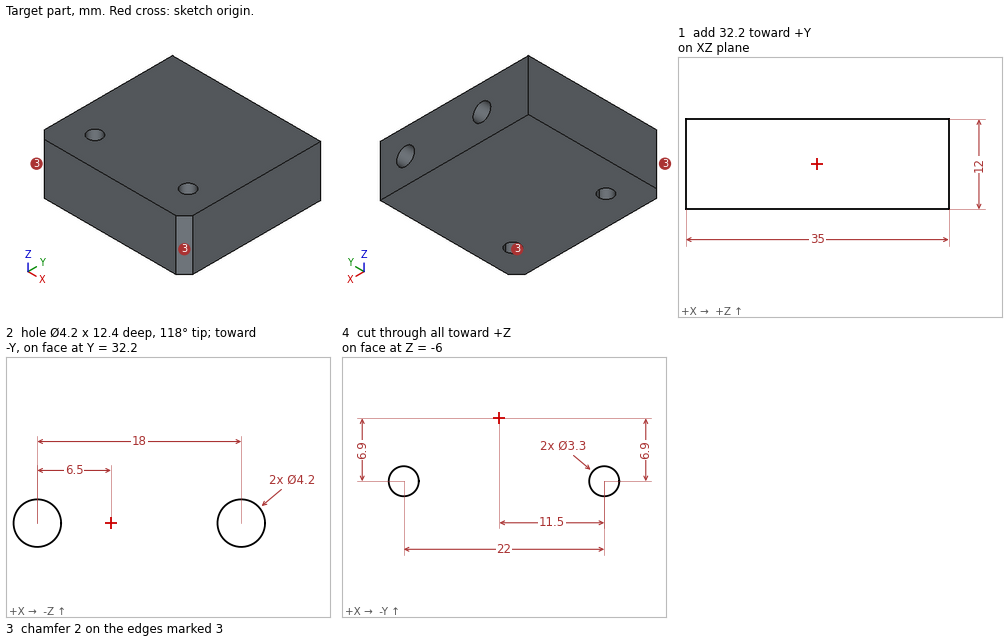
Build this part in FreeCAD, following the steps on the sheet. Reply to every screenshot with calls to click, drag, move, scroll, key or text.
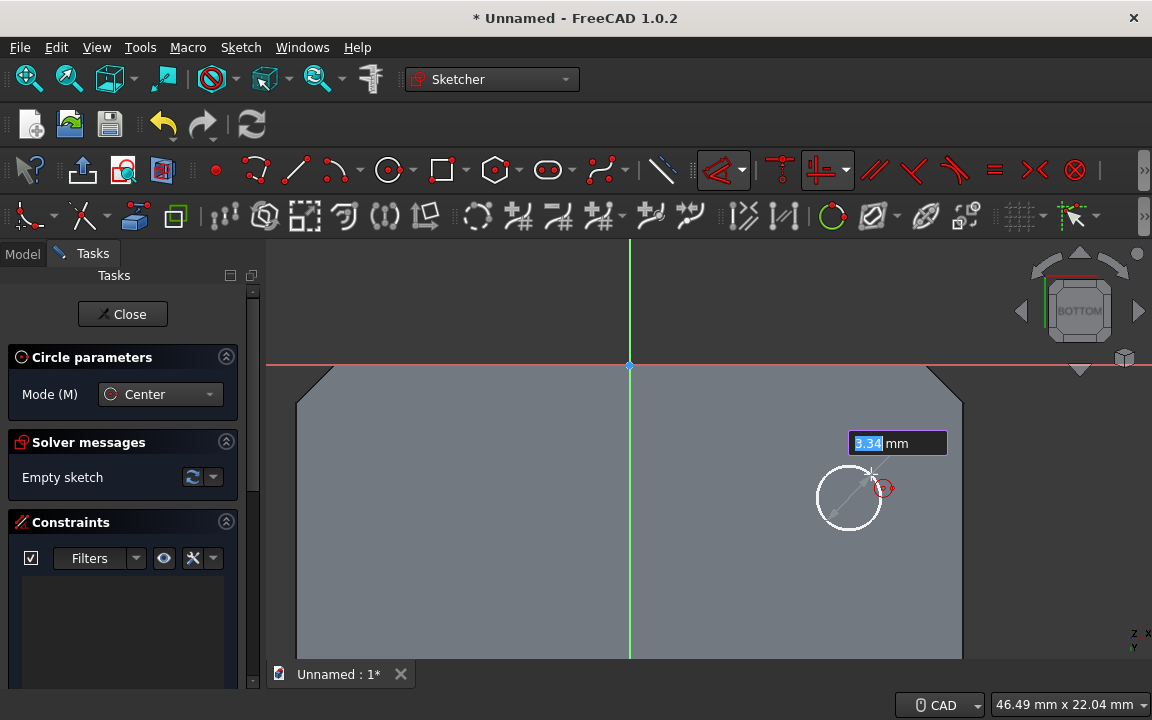
text(3.3)
key(Return)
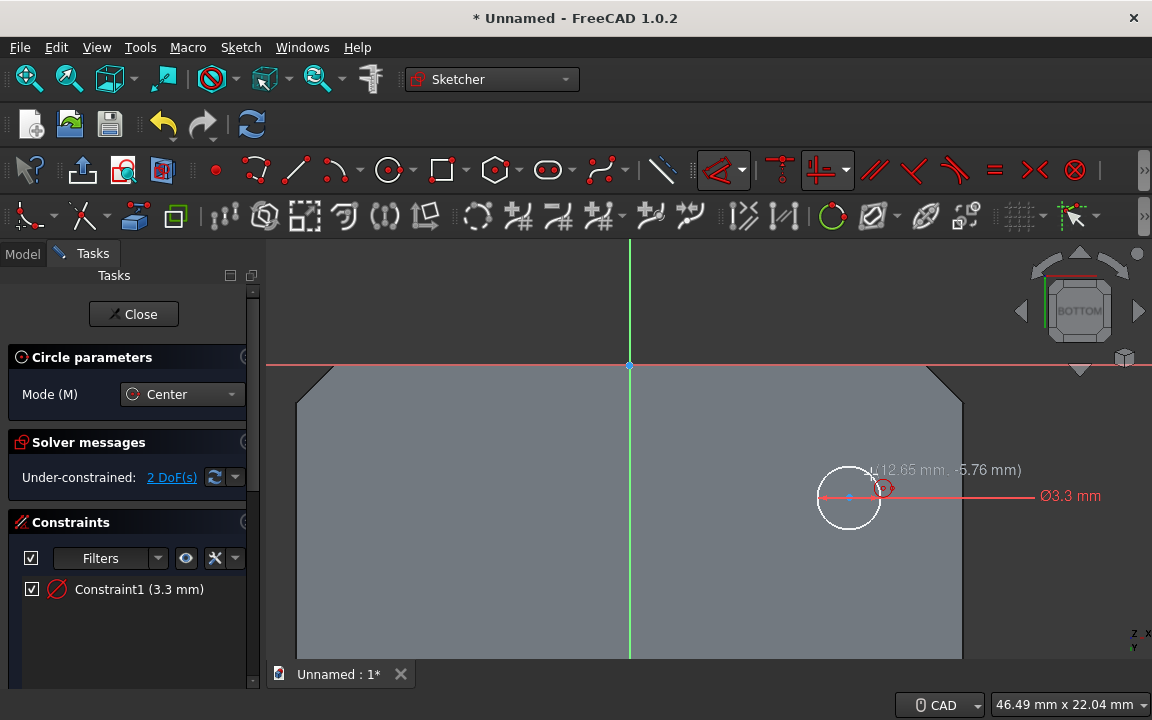
click(430, 497)
move(452, 474)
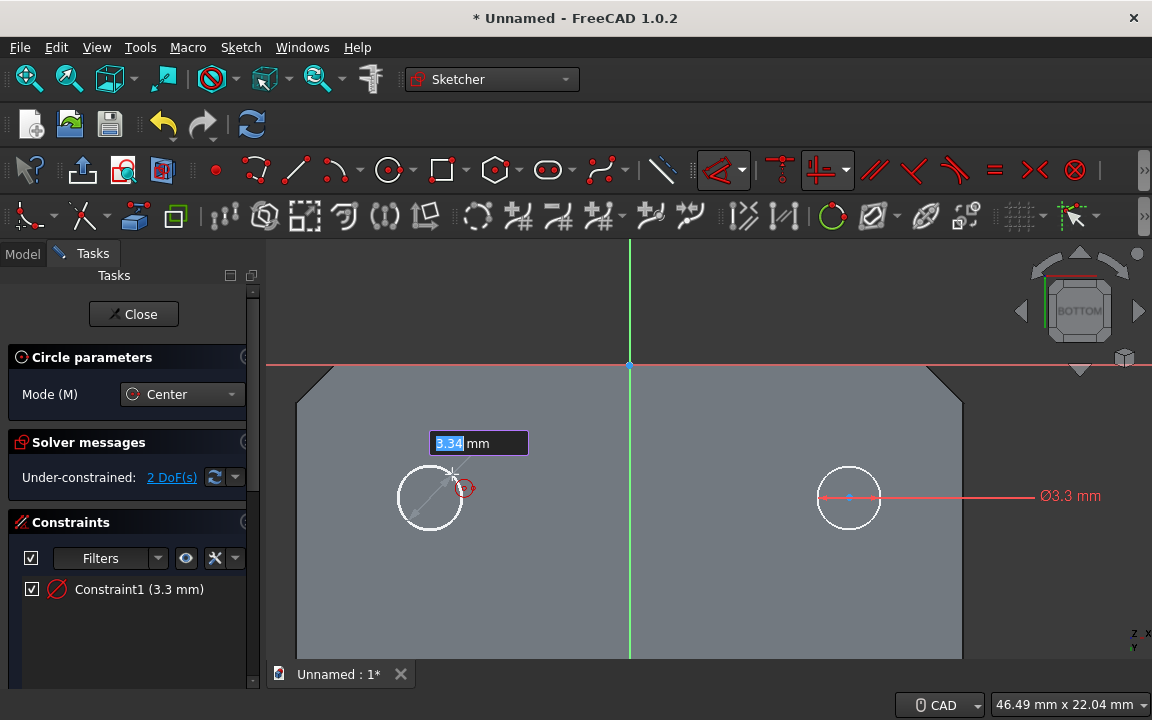
text(3.3)
key(Return)
key(Escape)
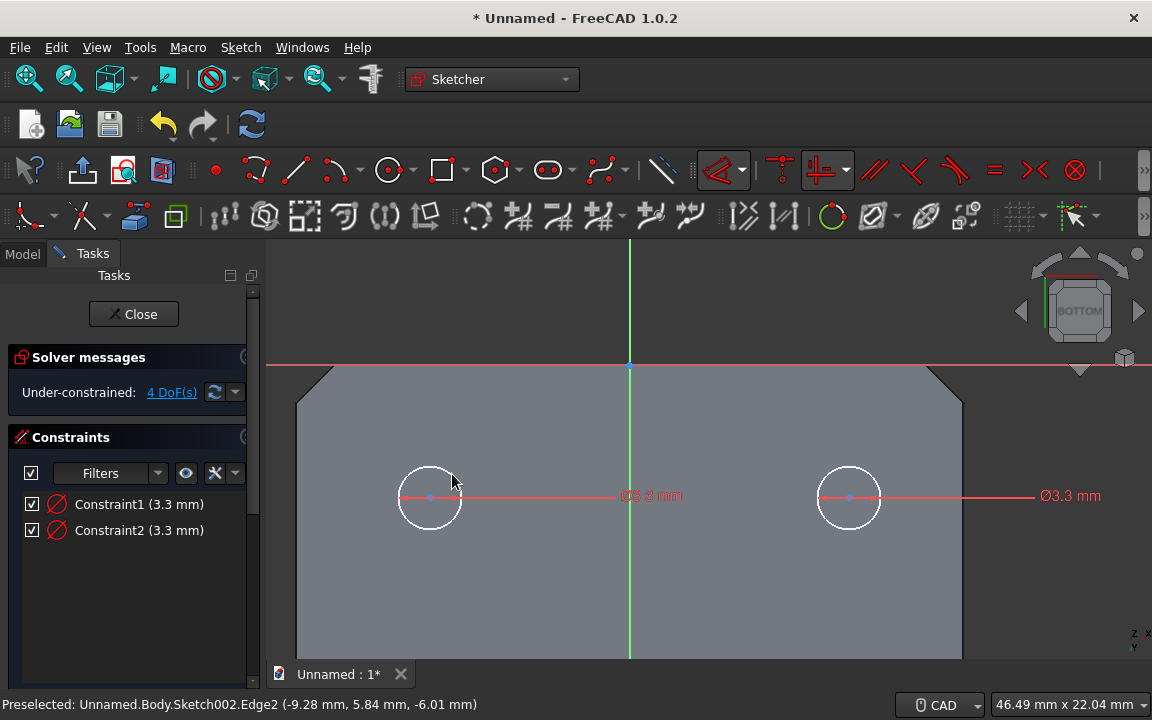
click(718, 170)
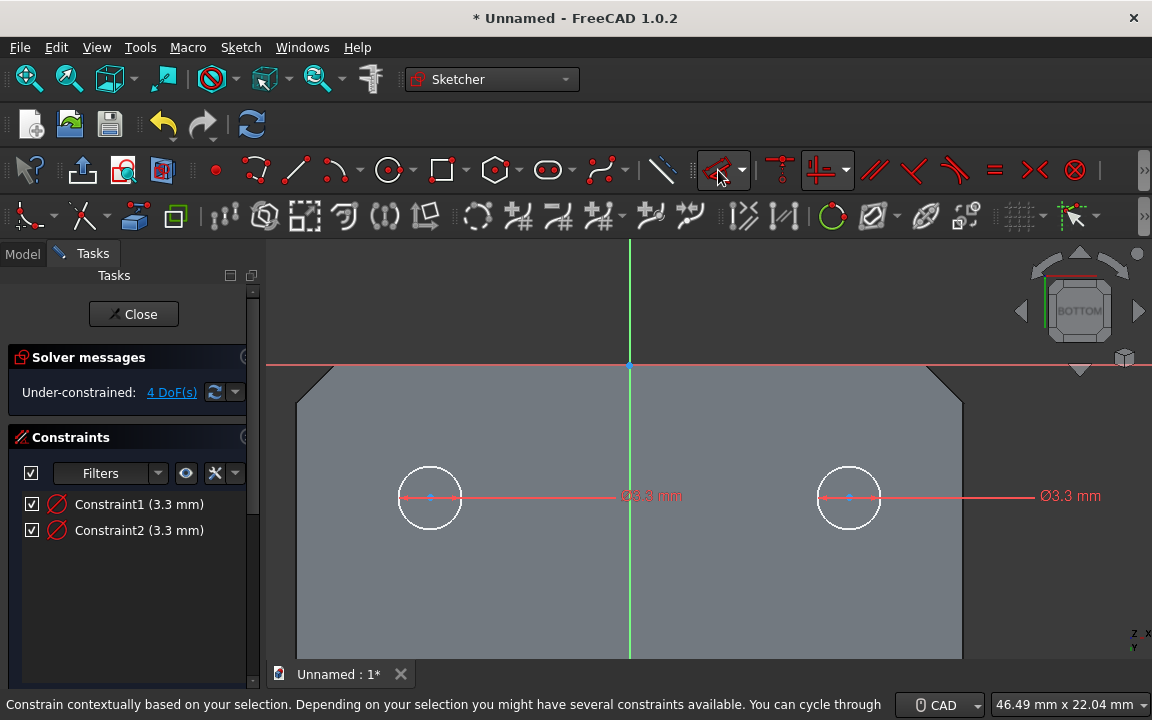
click(849, 498)
click(883, 432)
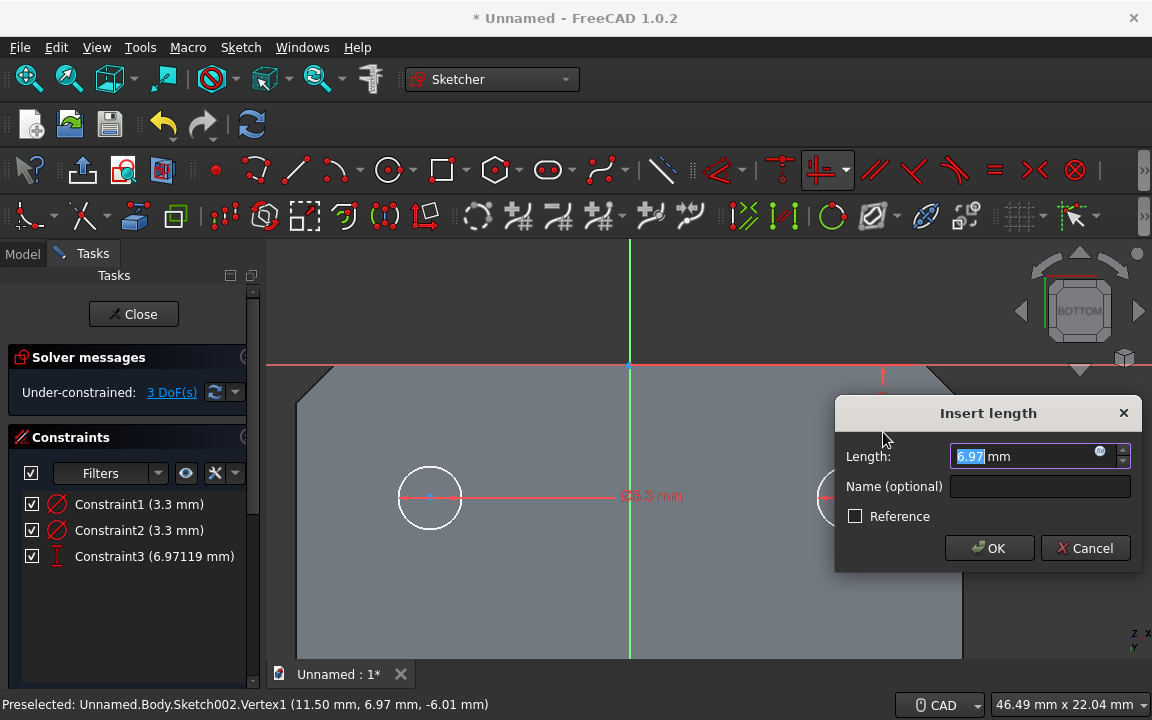
text(6.9)
key(Return)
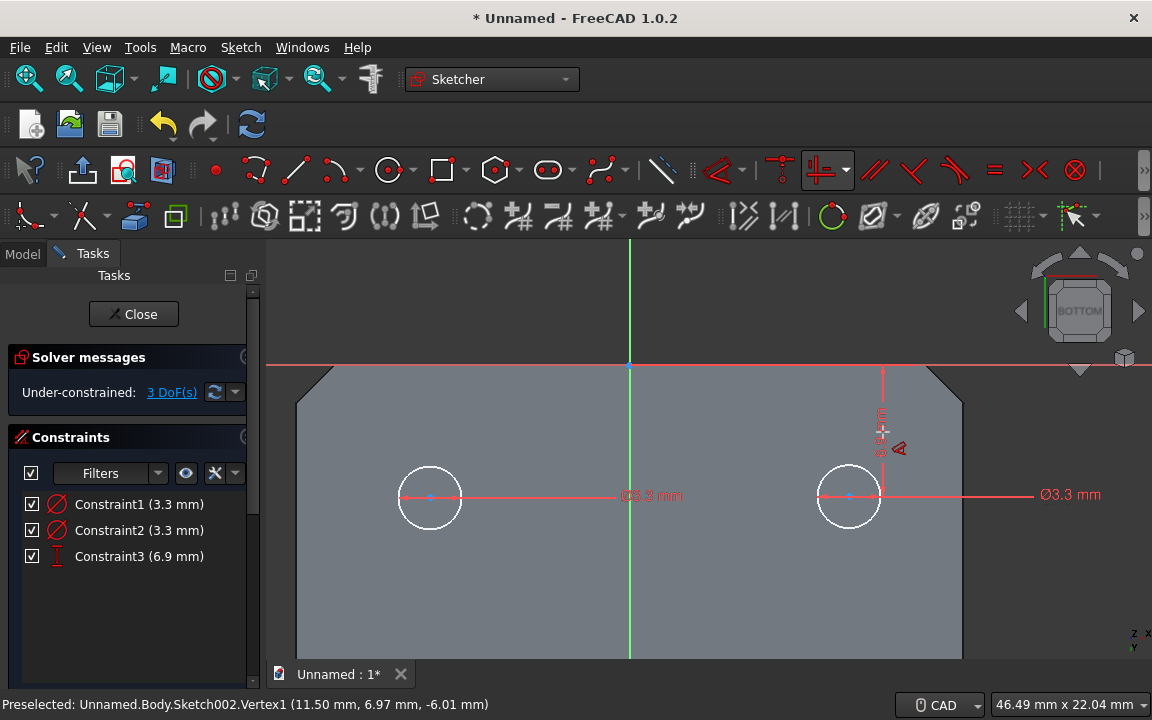
click(430, 498)
click(396, 432)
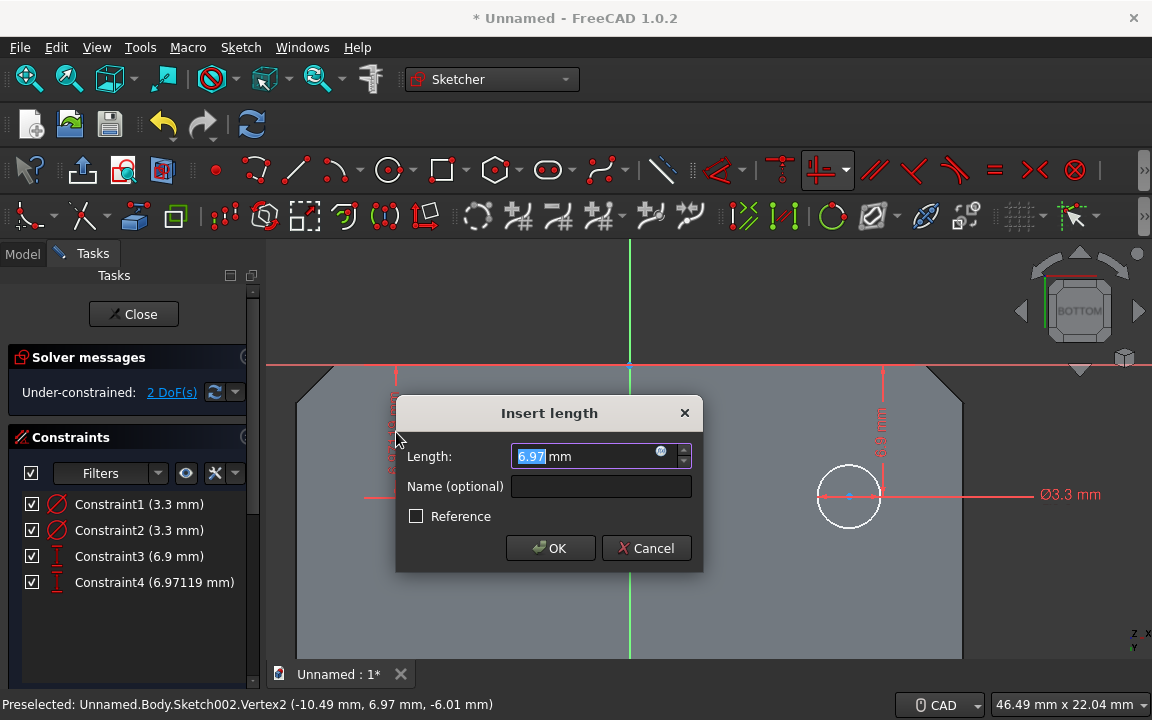
text(6.9)
key(Return)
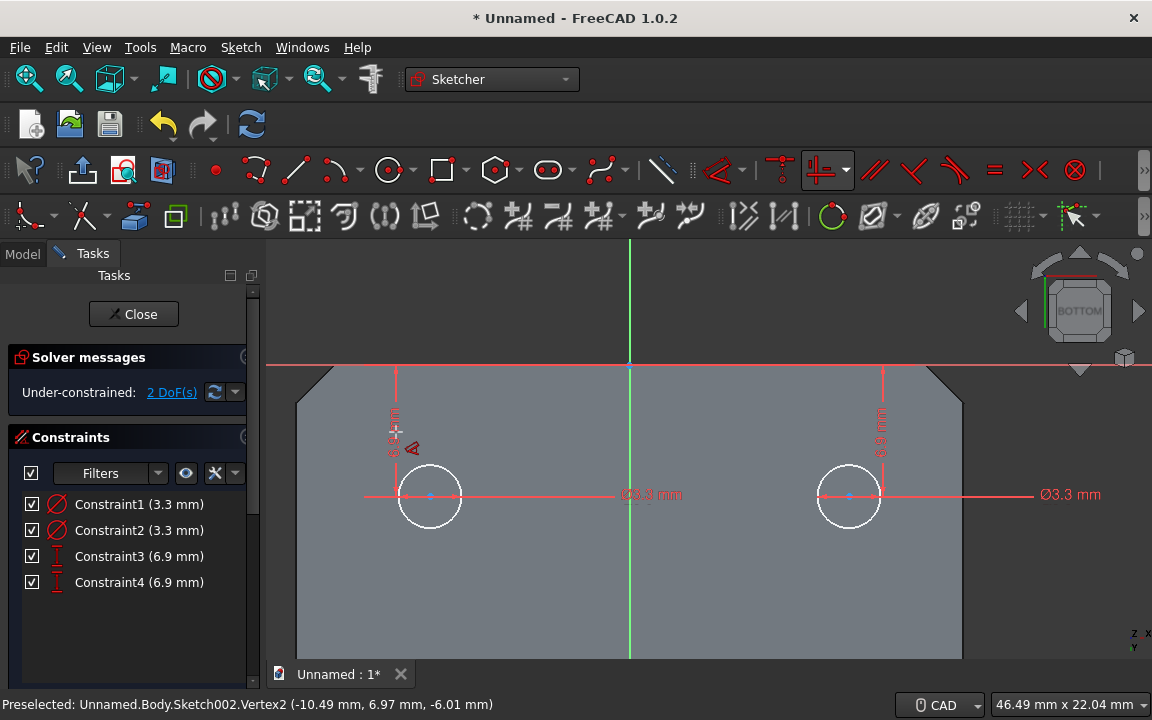
click(849, 497)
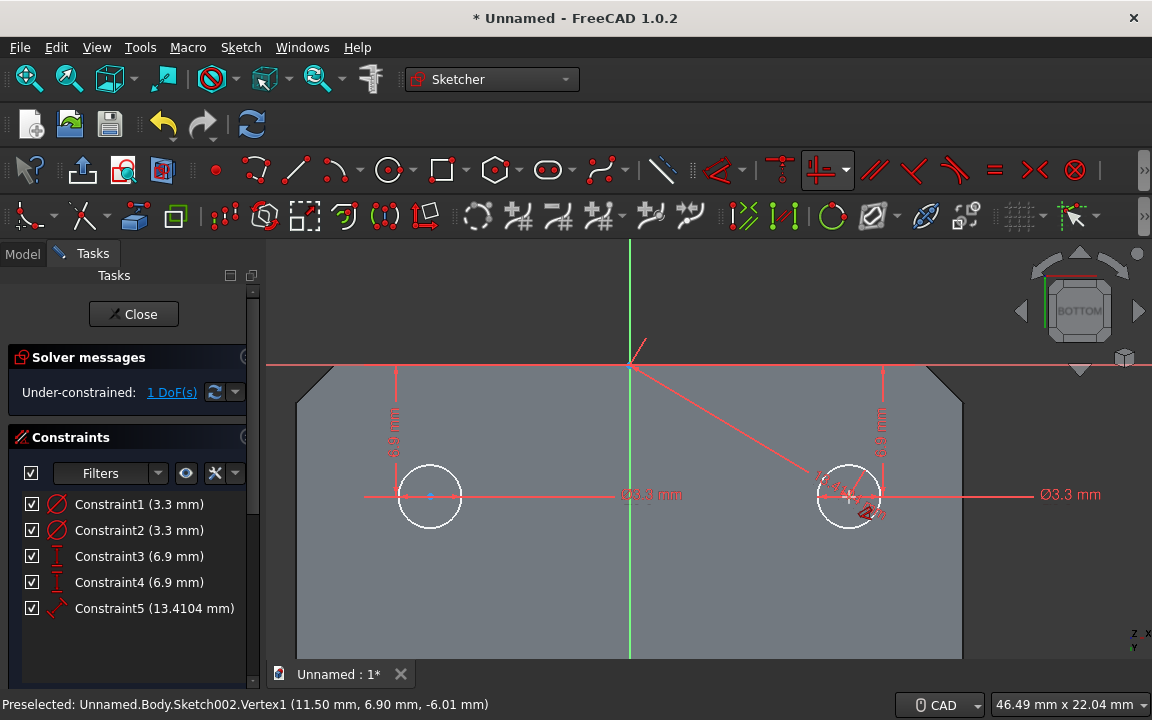
click(430, 497)
click(543, 531)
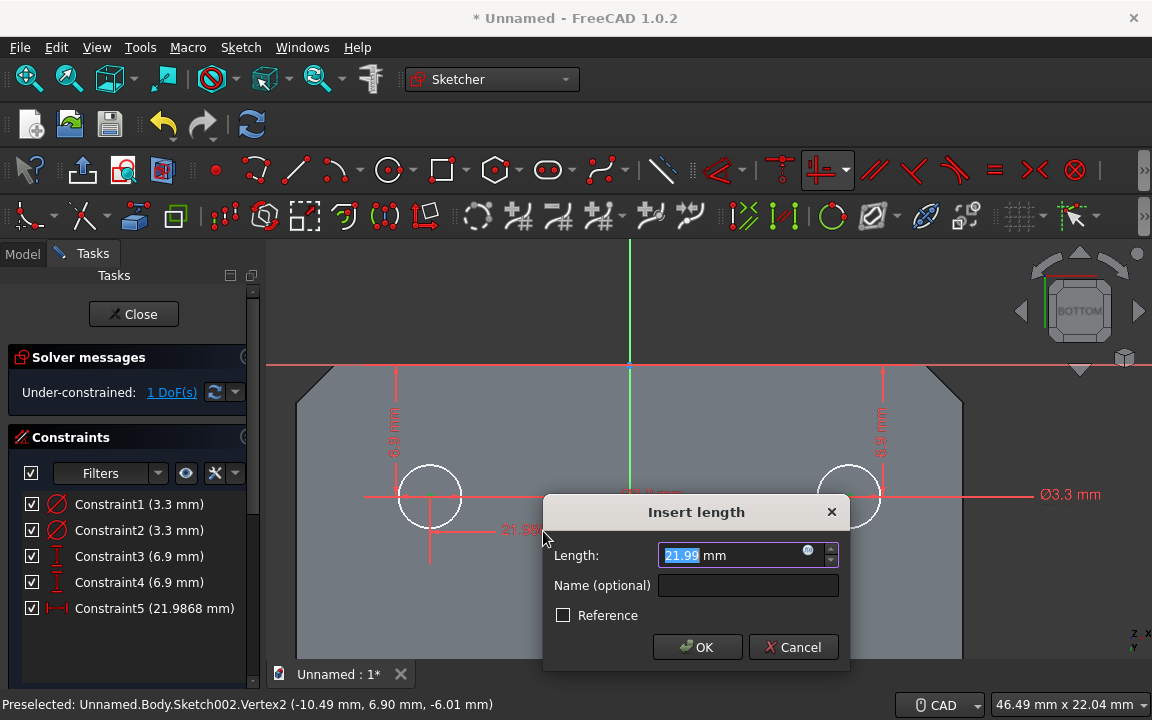
text(22)
key(Return)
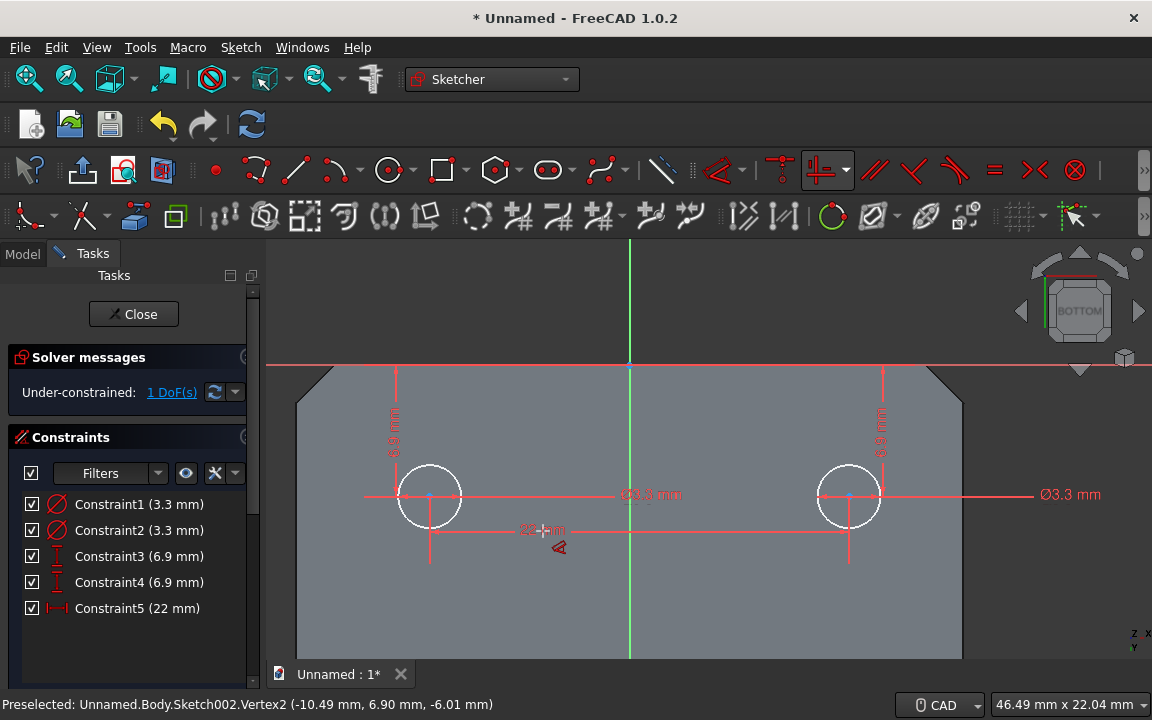
click(849, 497)
click(739, 331)